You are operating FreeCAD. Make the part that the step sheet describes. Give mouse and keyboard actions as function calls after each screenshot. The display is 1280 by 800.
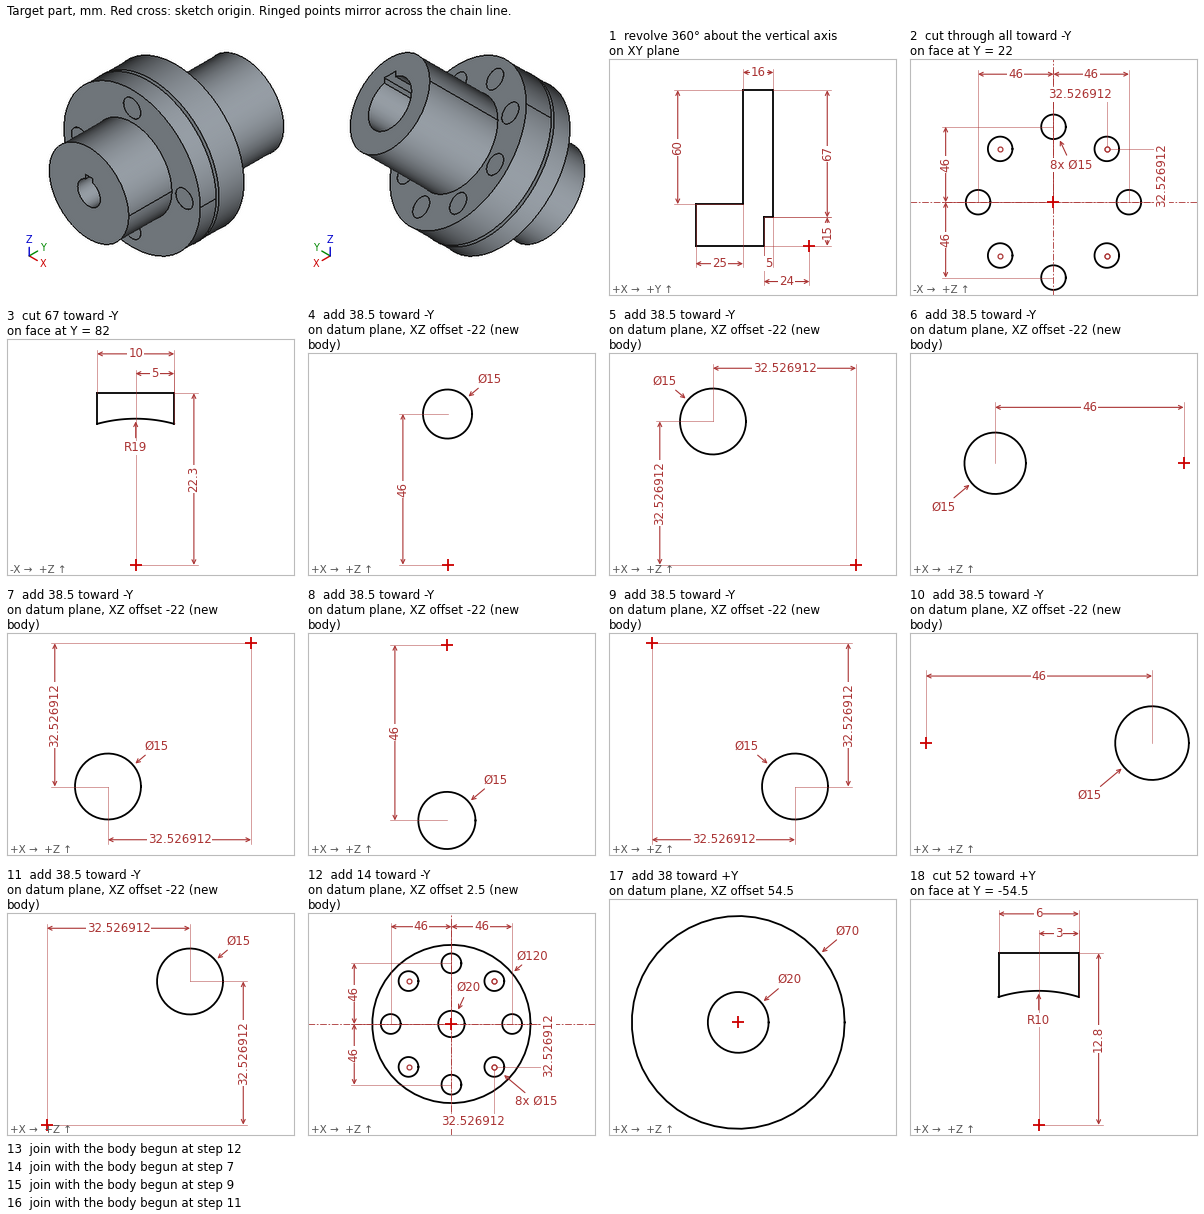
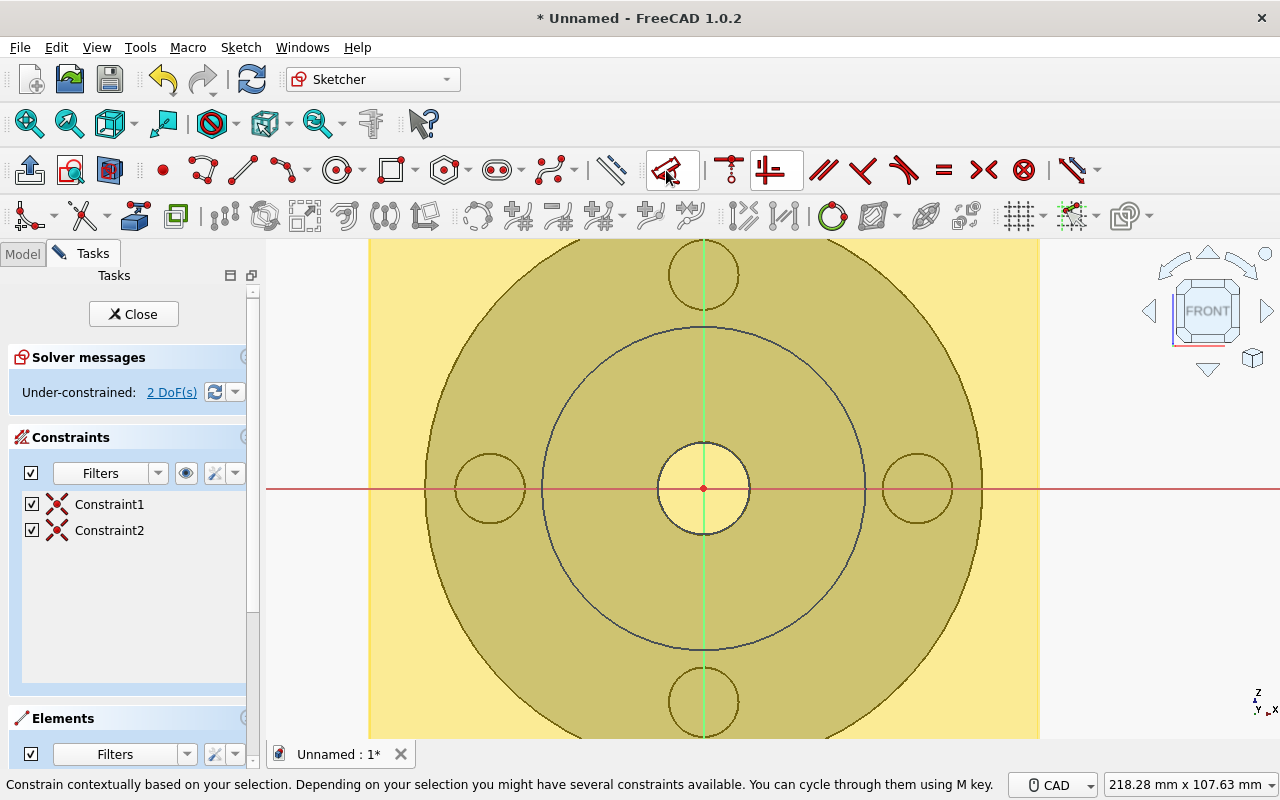
click(818, 374)
click(841, 351)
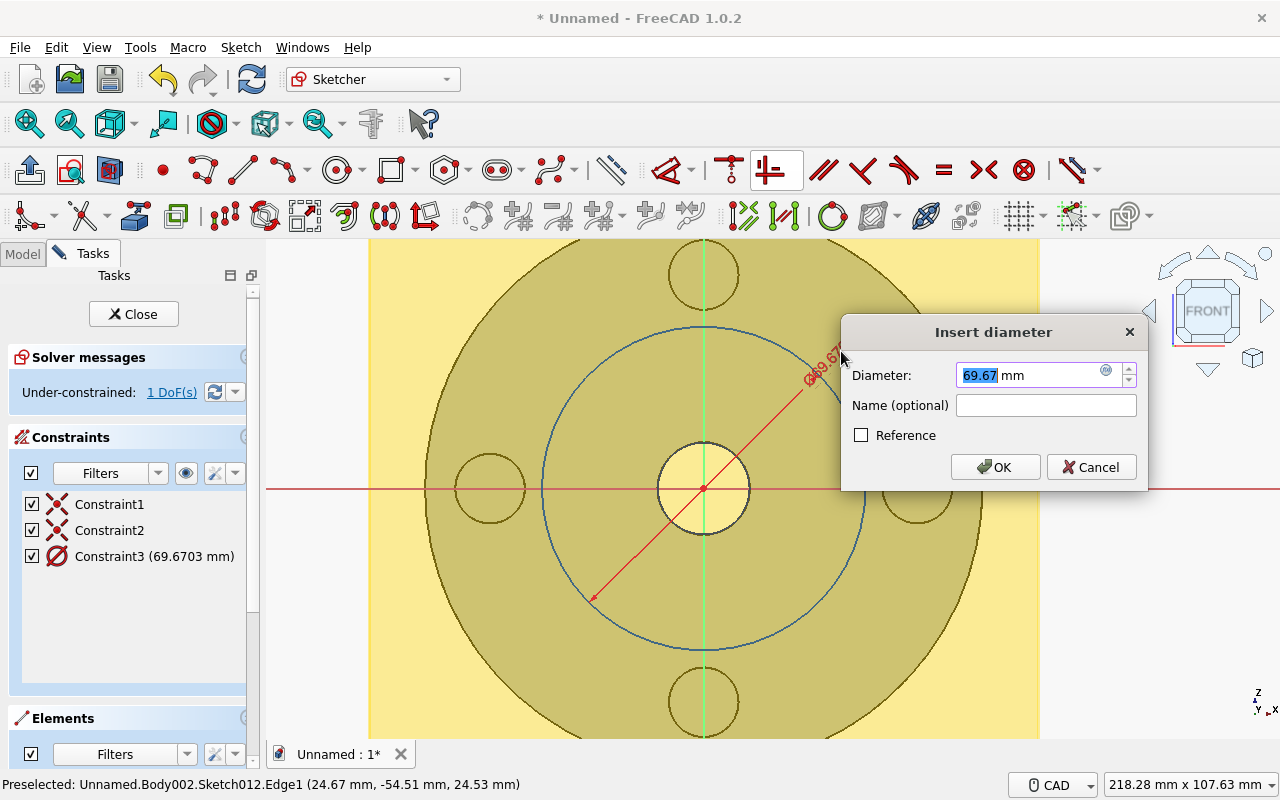
text(70)
key(Return)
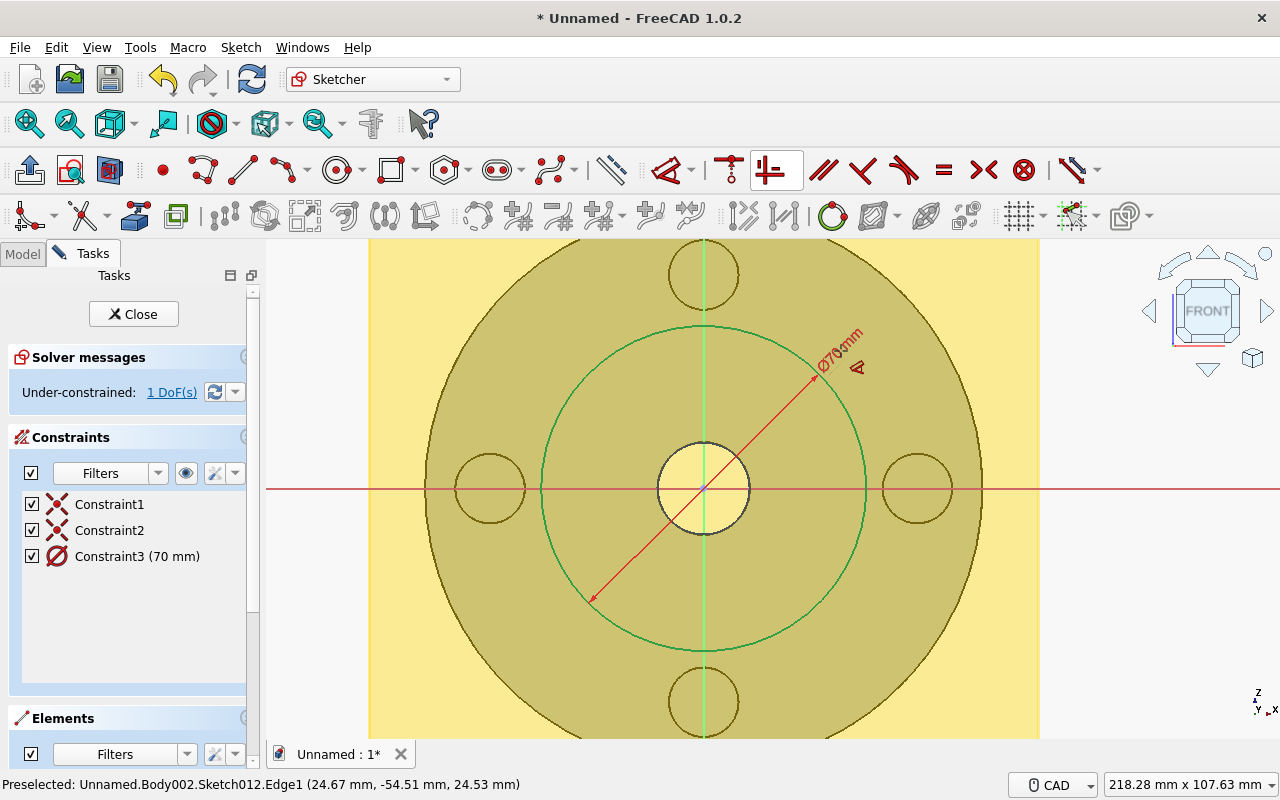
click(736, 456)
click(759, 433)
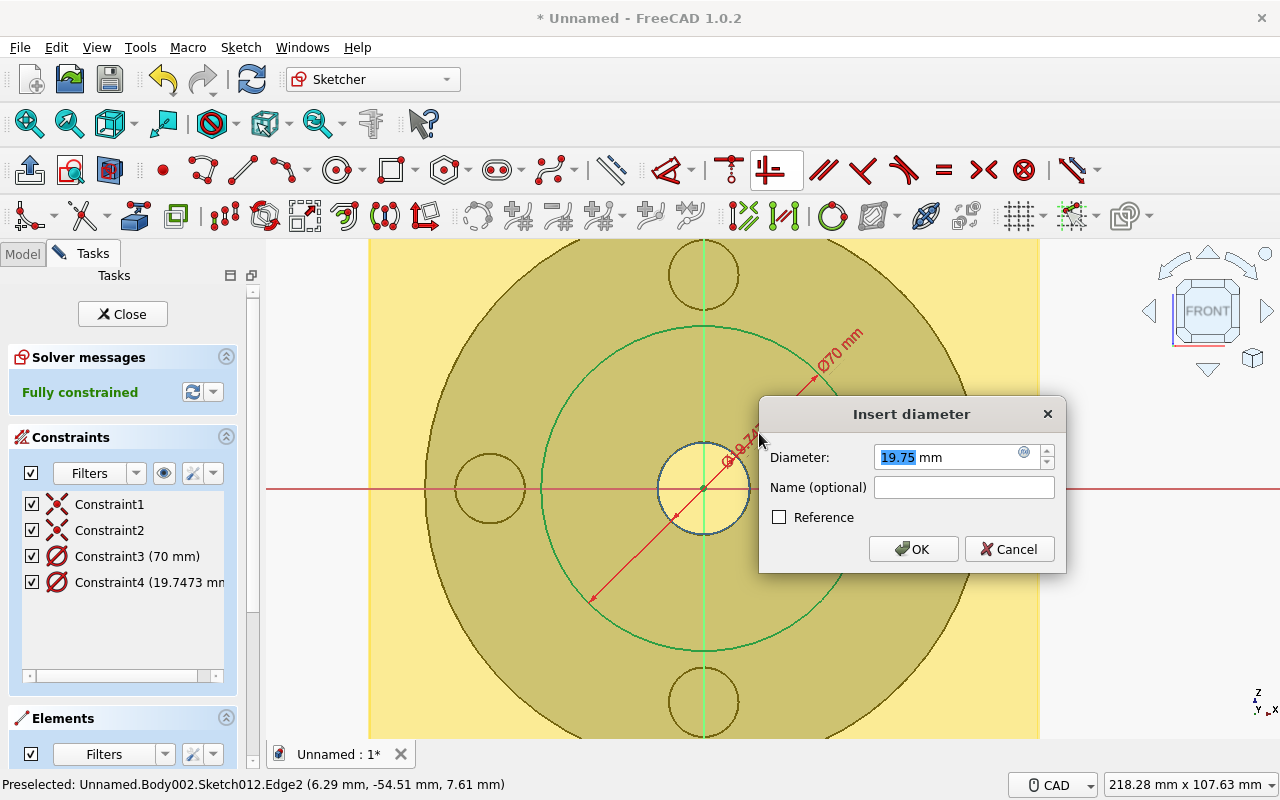
text(20)
key(Return)
key(Escape)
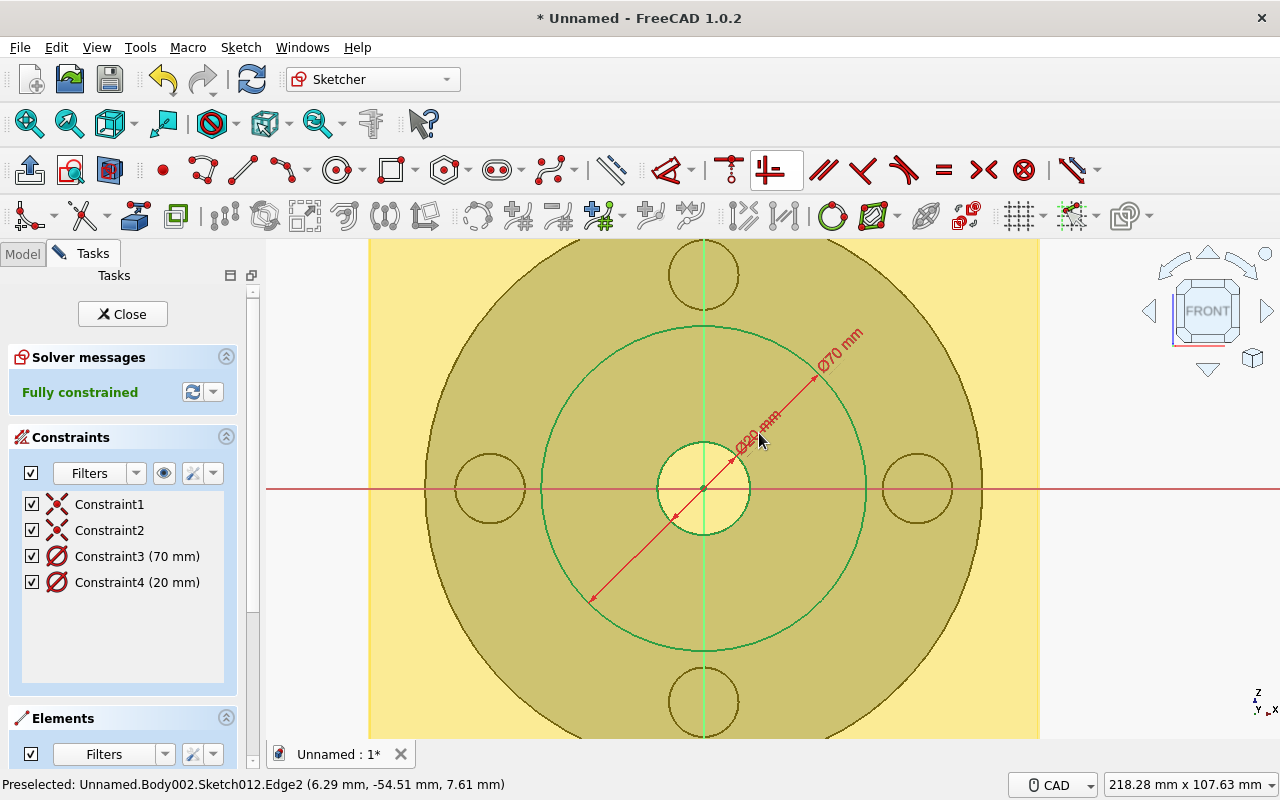
click(123, 314)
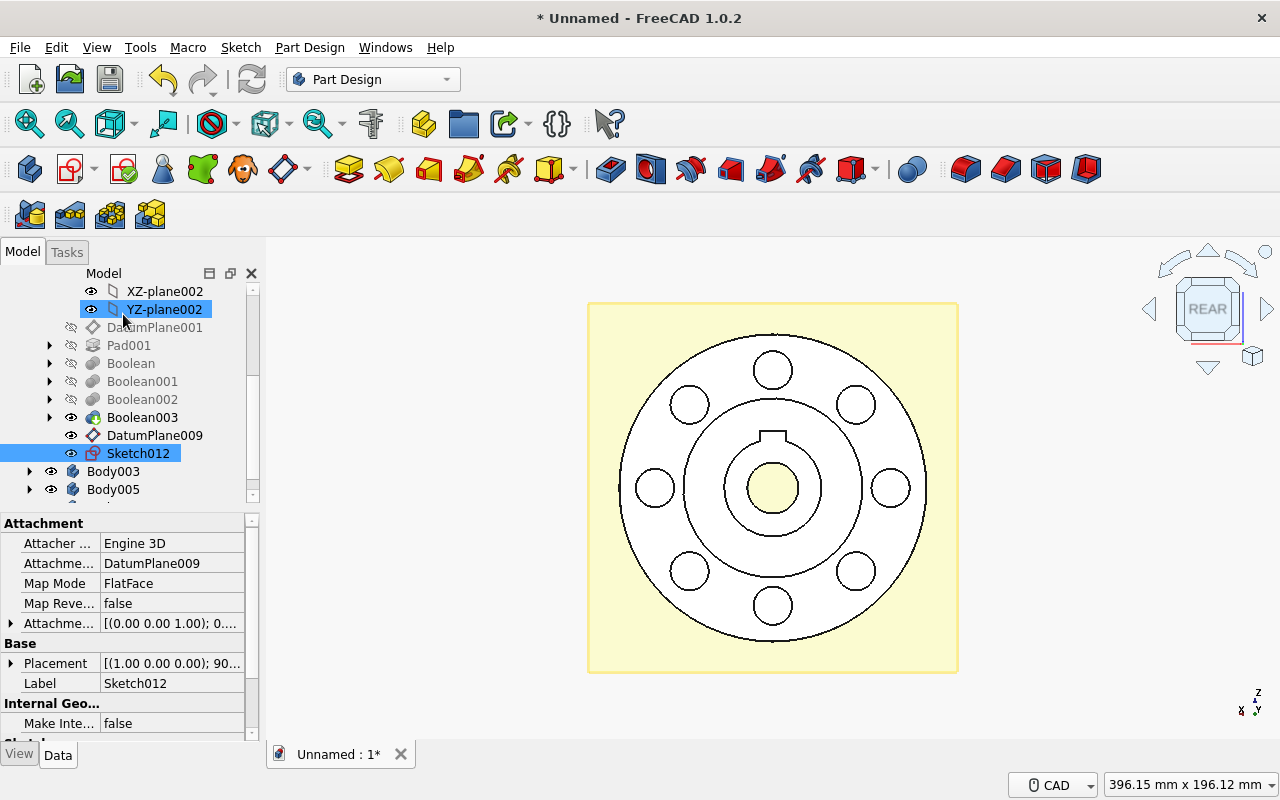
click(350, 170)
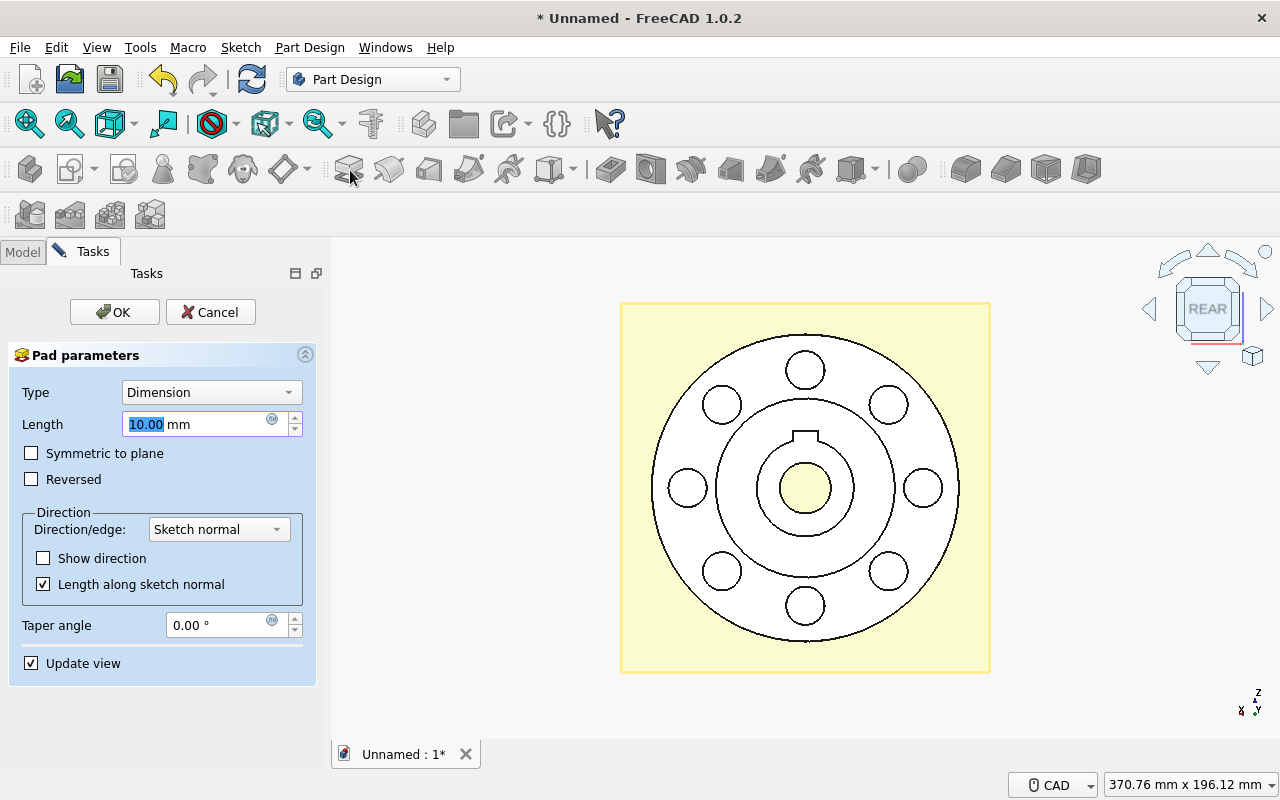
text(38)
key(Tab)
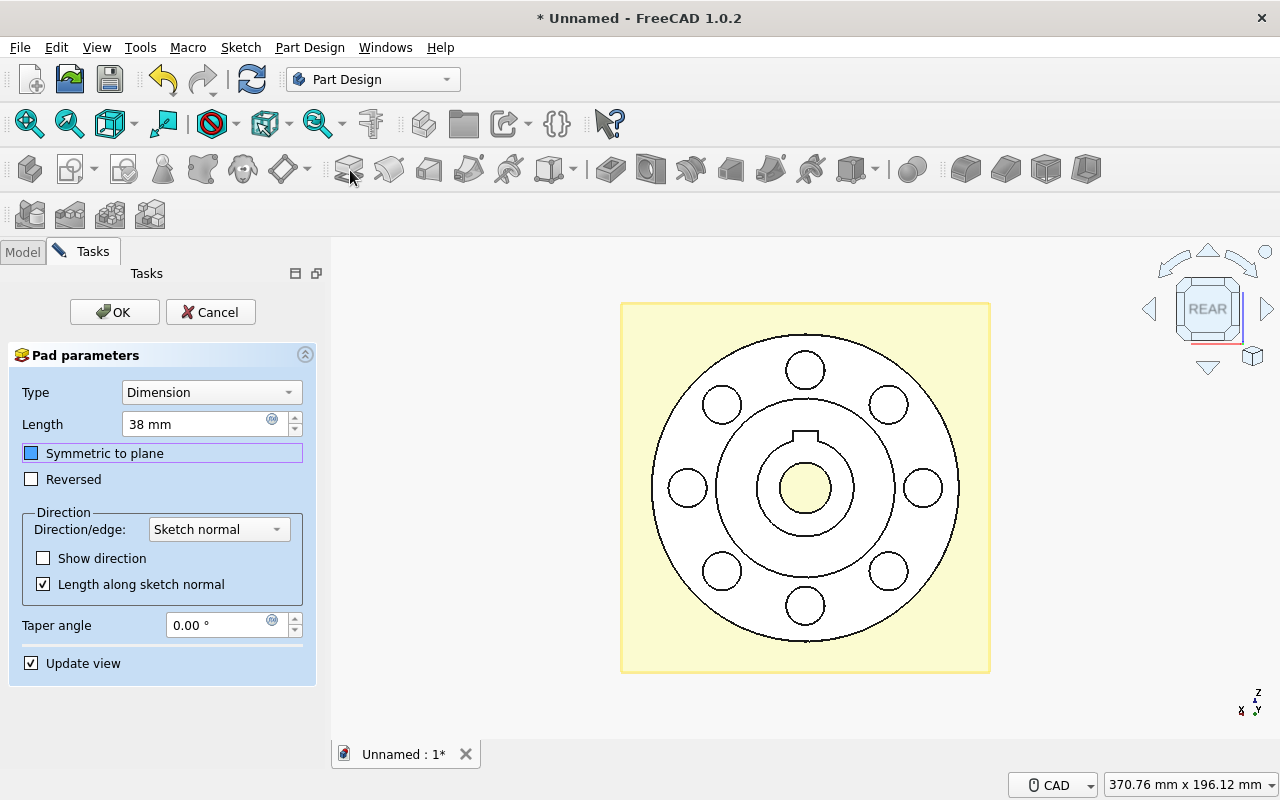
click(30, 479)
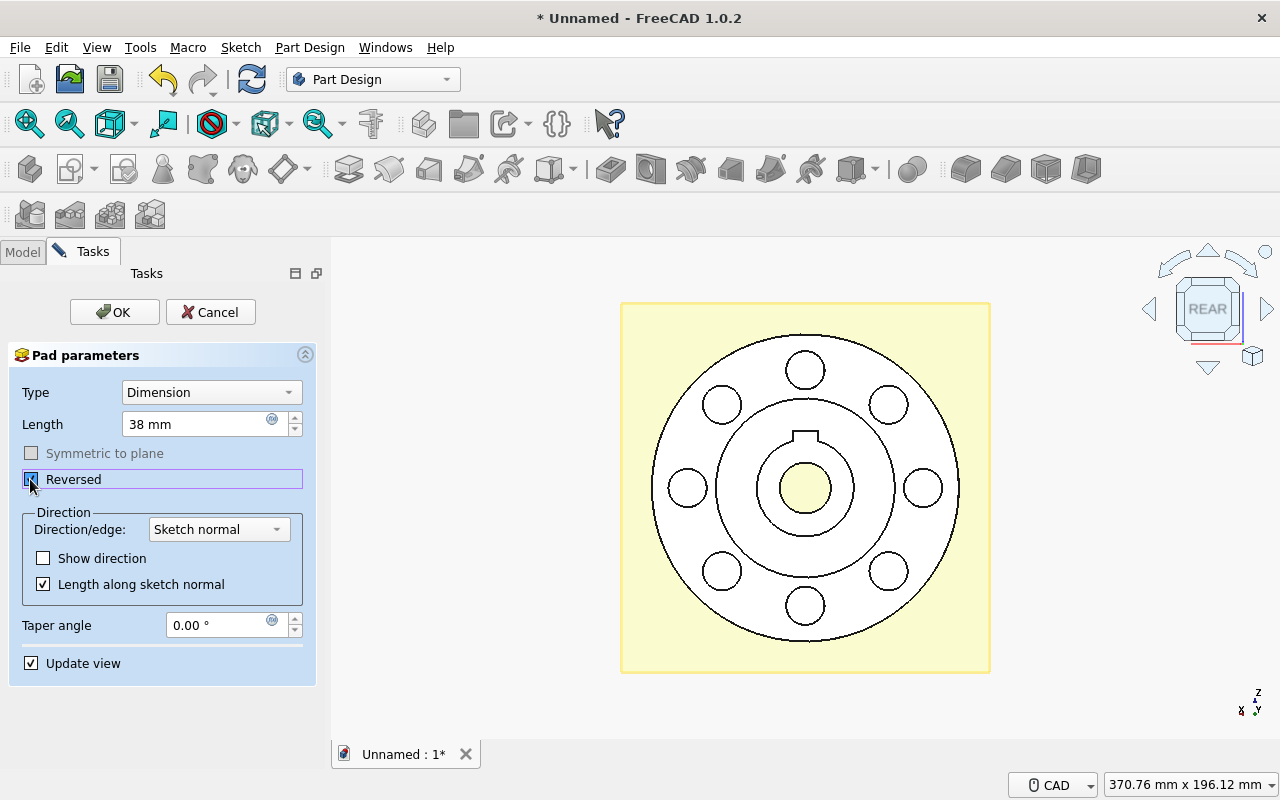
click(115, 312)